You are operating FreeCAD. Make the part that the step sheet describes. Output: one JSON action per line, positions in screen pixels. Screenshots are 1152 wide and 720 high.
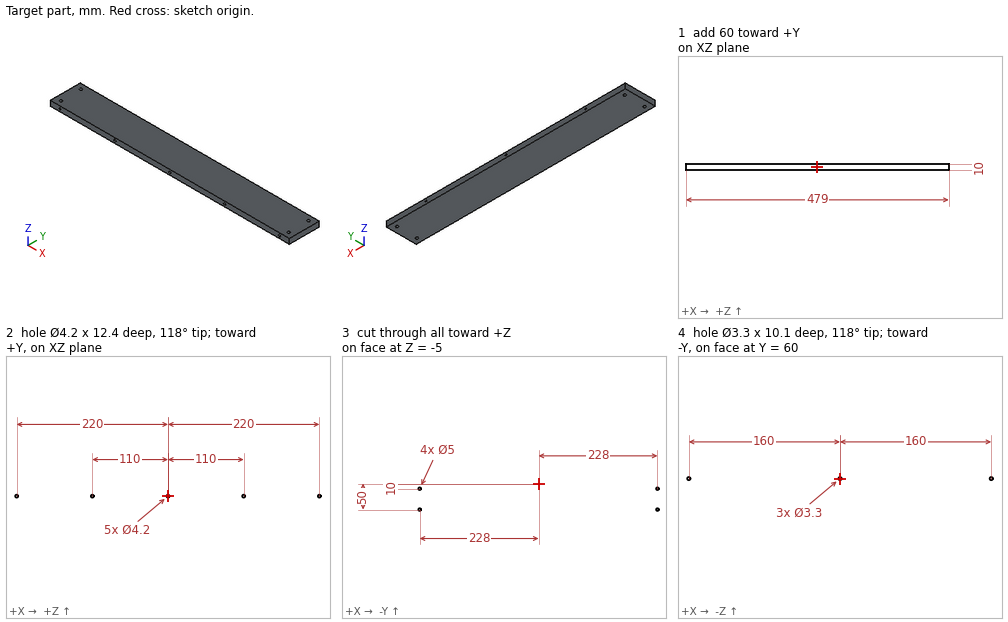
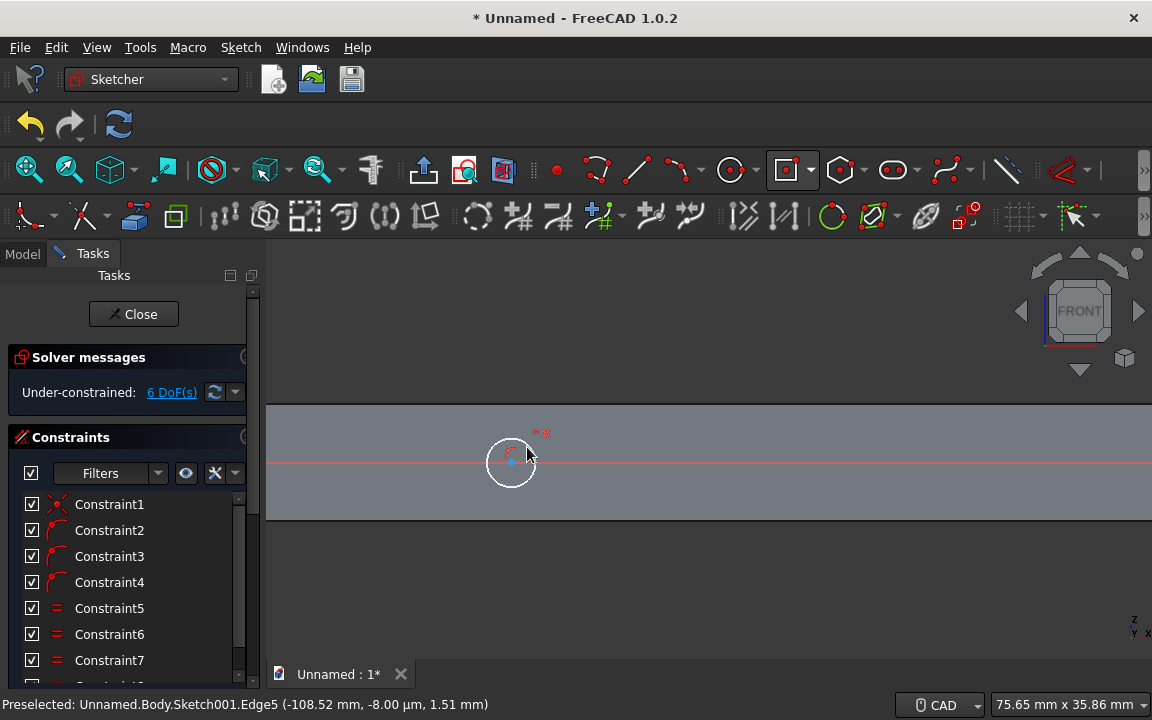
{"action": "scroll", "coordinate": [525, 448], "scroll_direction": "down", "scroll_amount": 12}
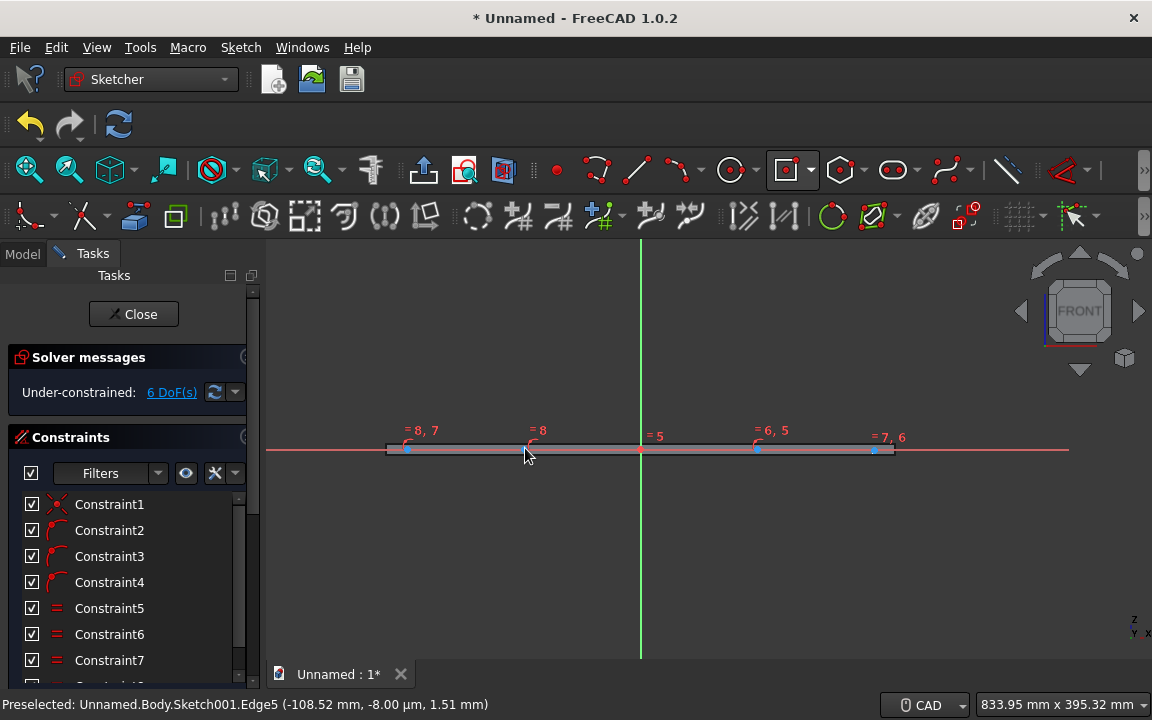
{"action": "left_click", "coordinate": [874, 451]}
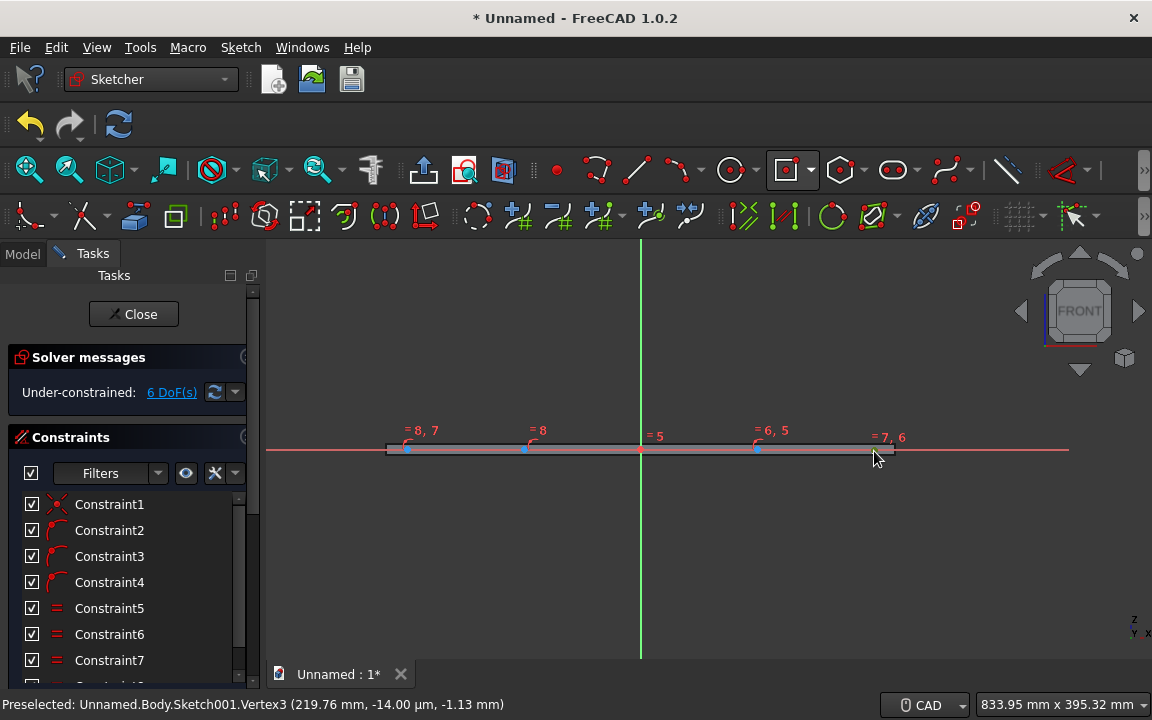
{"action": "left_click", "coordinate": [344, 450]}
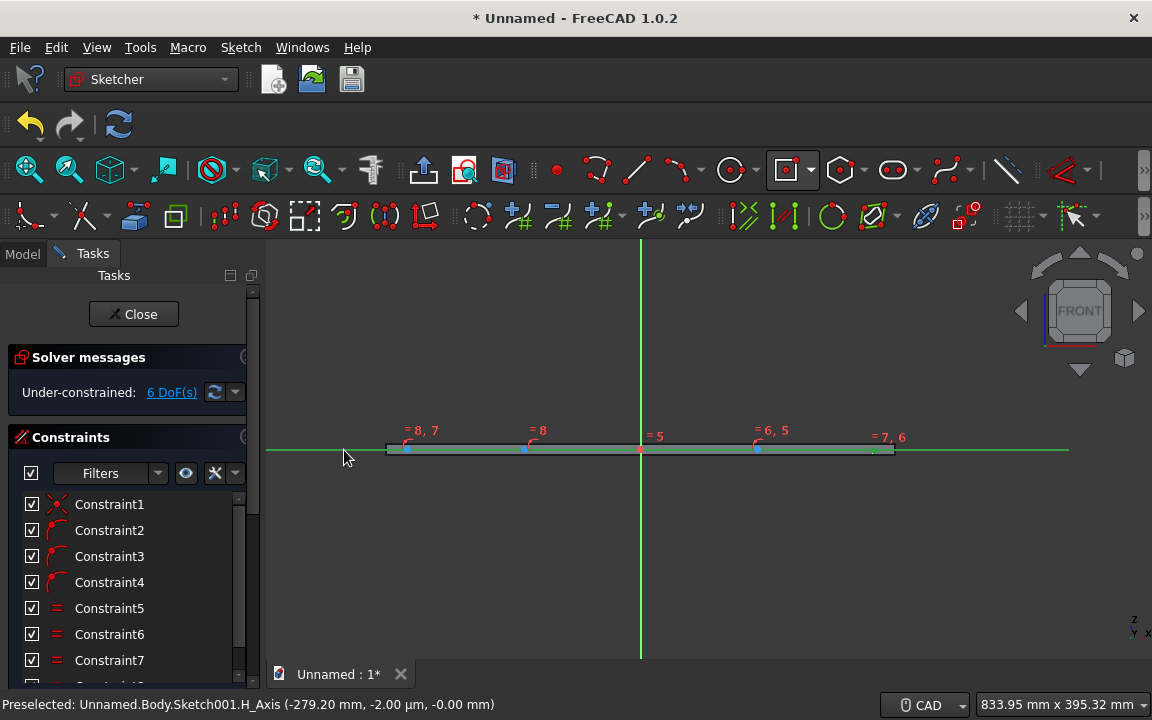
{"action": "key", "text": "c"}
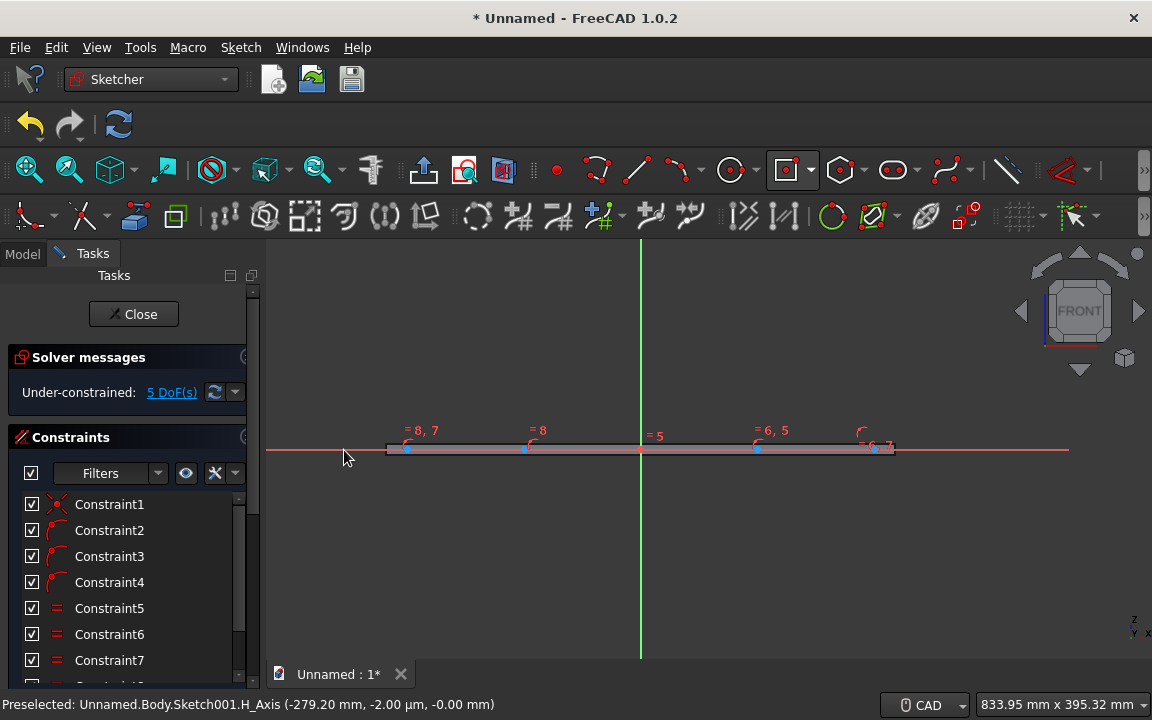
{"action": "key", "text": "d"}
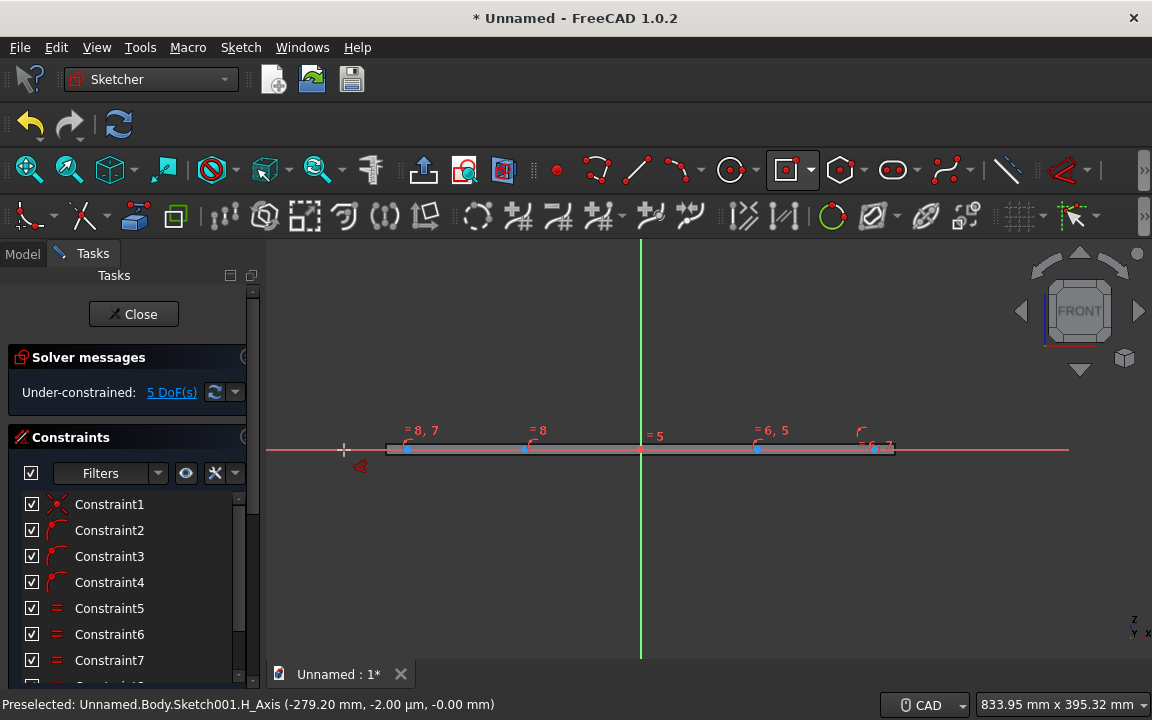
{"action": "scroll", "coordinate": [642, 448], "scroll_direction": "up", "scroll_amount": 11}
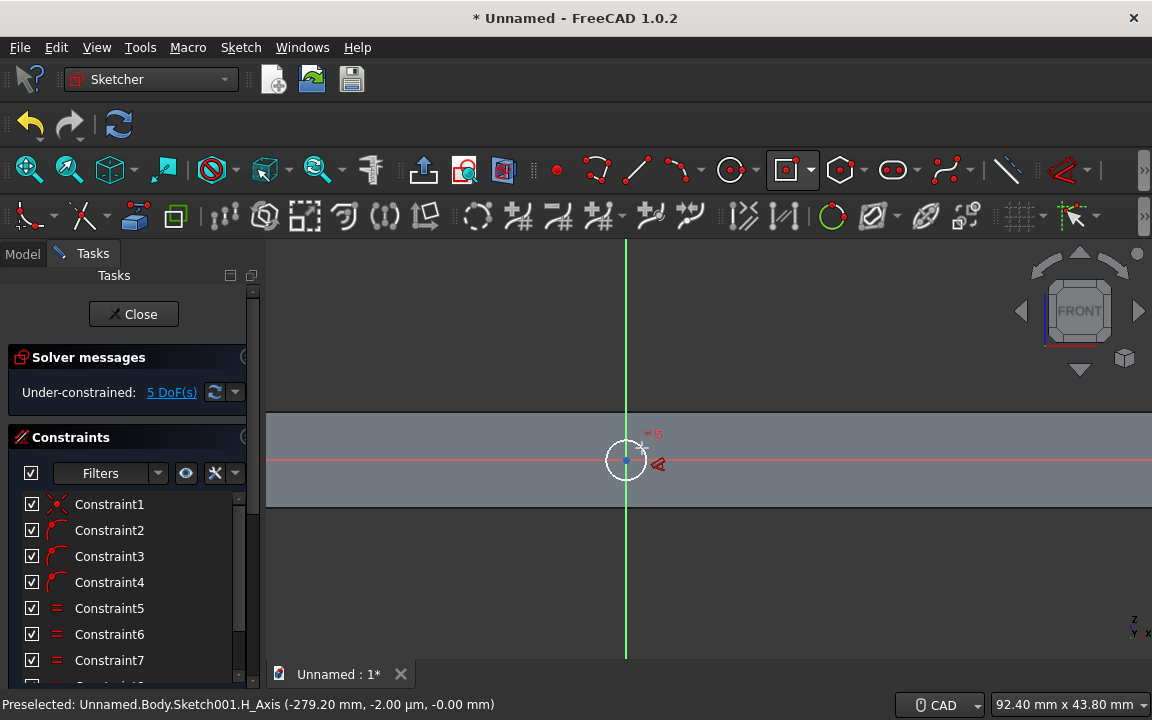
{"action": "left_click", "coordinate": [640, 446]}
{"action": "left_click", "coordinate": [662, 423]}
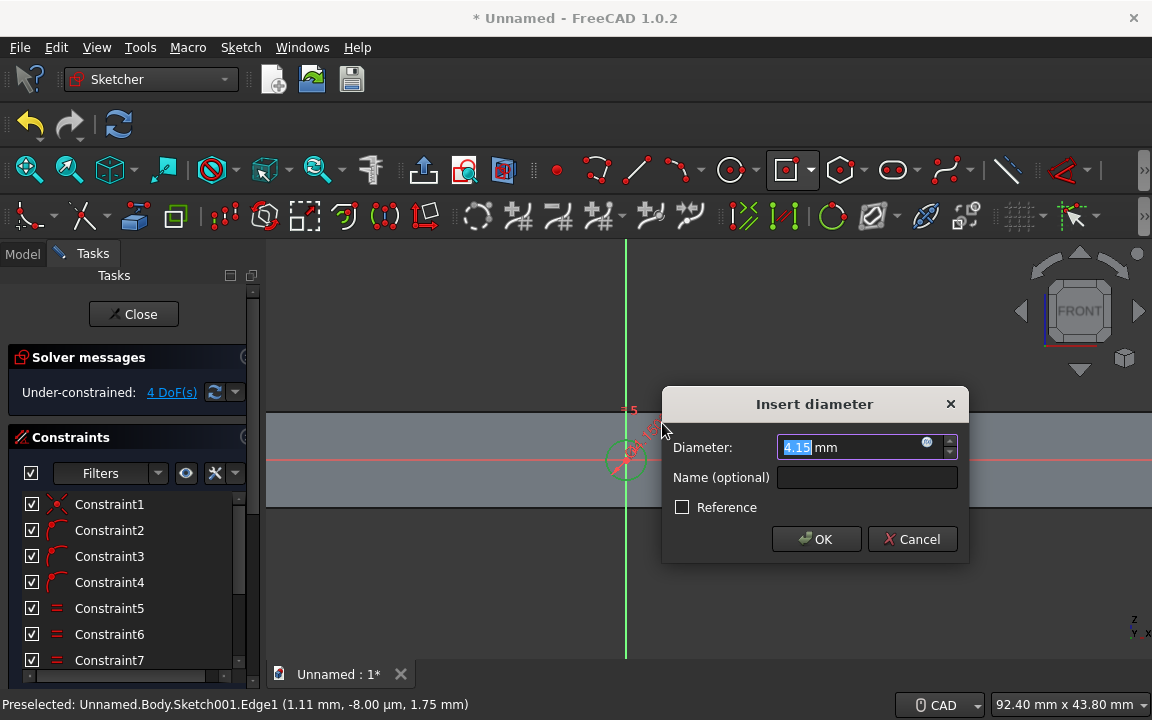
{"action": "type", "text": "4.2"}
{"action": "key", "text": "Return"}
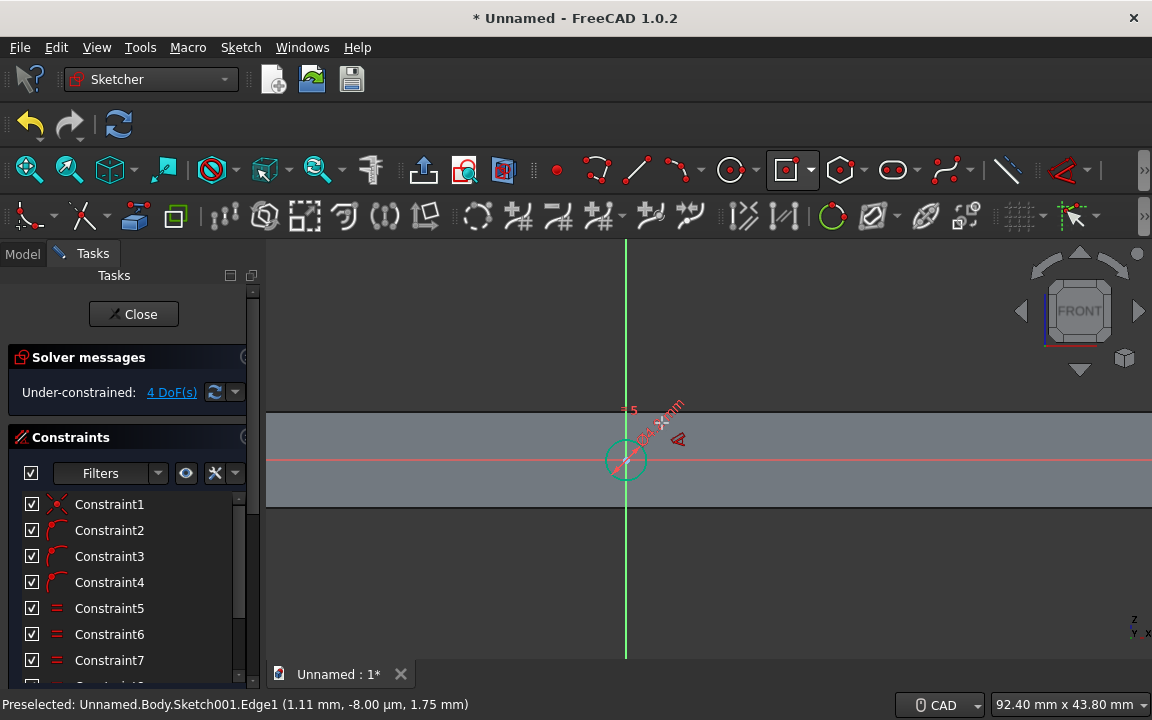
{"action": "scroll", "coordinate": [642, 448], "scroll_direction": "down", "scroll_amount": 11}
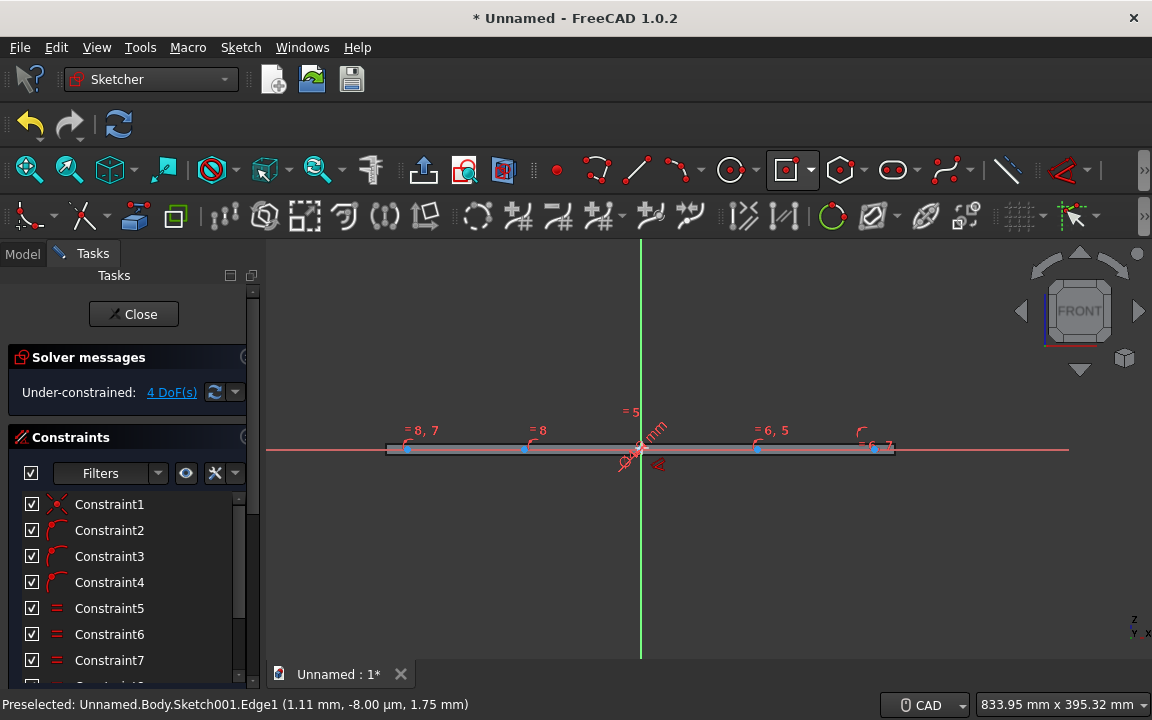
{"action": "left_click", "coordinate": [757, 450]}
{"action": "left_click", "coordinate": [699, 484]}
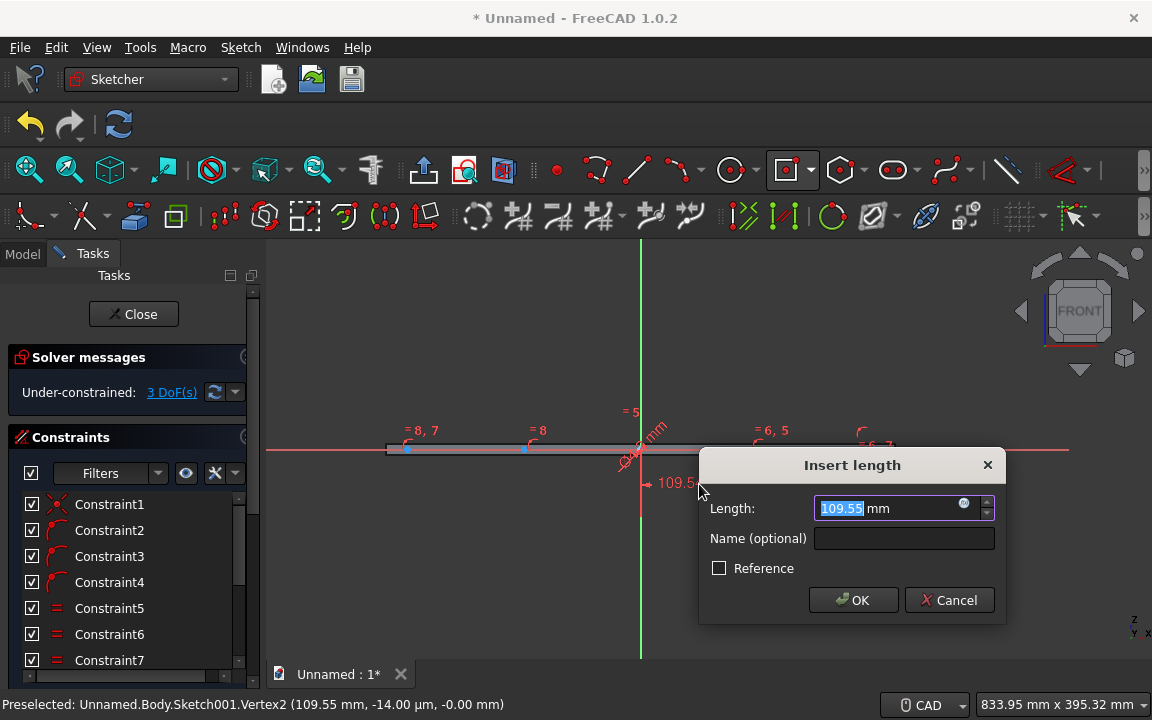
{"action": "type", "text": "110"}
{"action": "key", "text": "Return"}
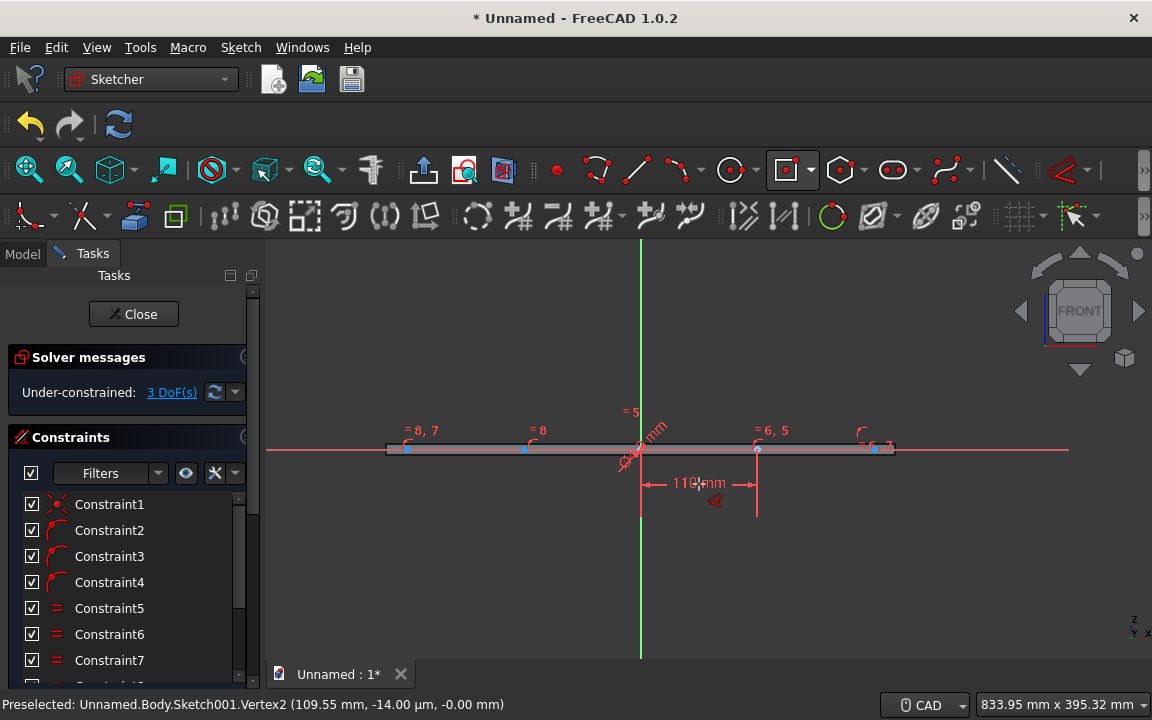
{"action": "left_click", "coordinate": [874, 450]}
{"action": "left_click", "coordinate": [811, 484]}